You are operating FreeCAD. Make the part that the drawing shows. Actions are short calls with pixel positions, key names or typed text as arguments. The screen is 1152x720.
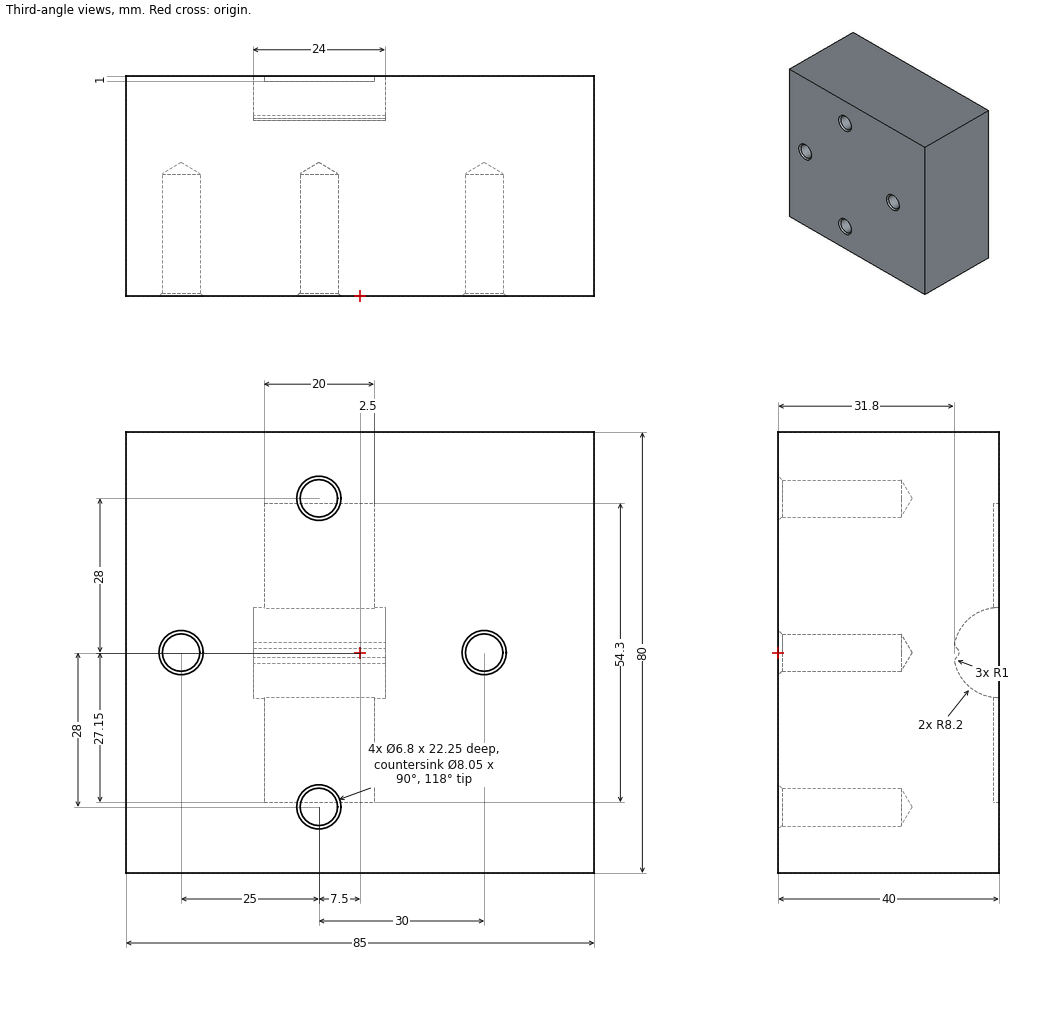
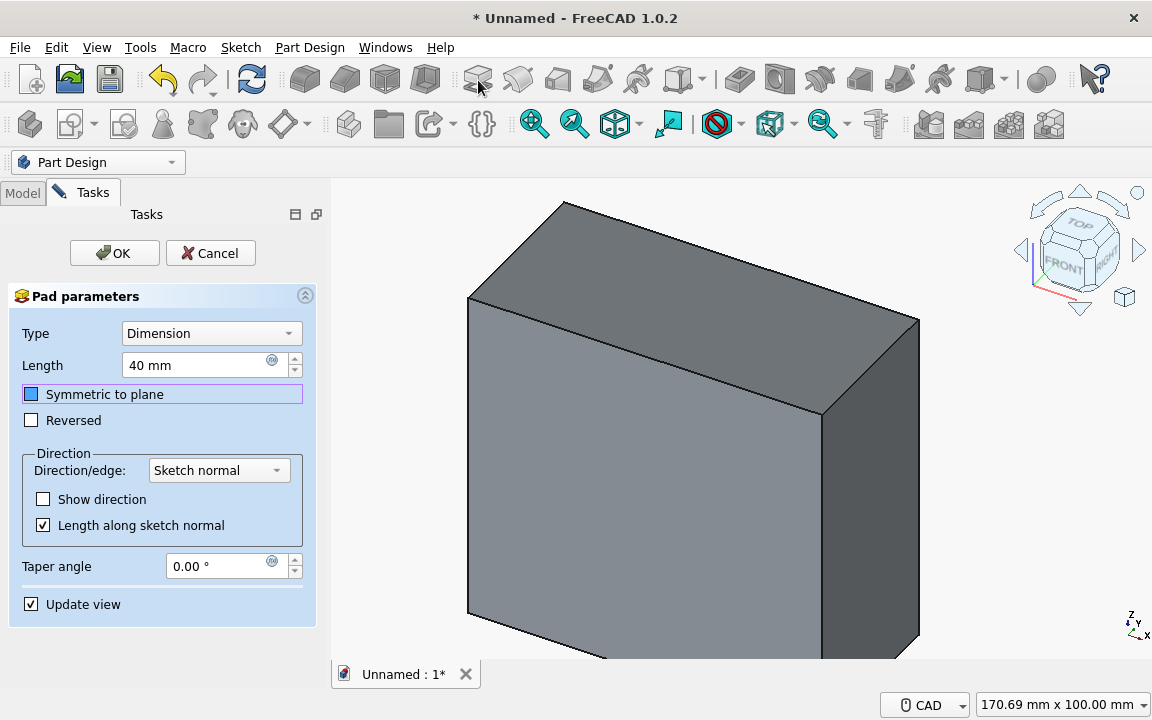
click(30, 420)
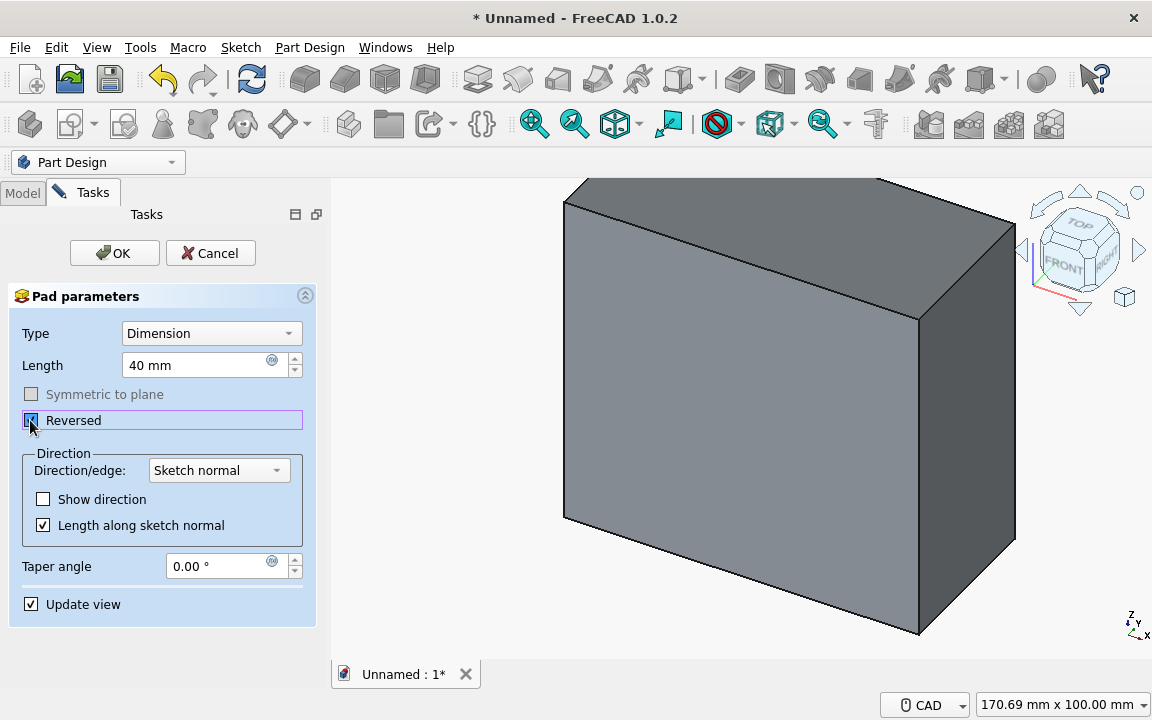
click(115, 253)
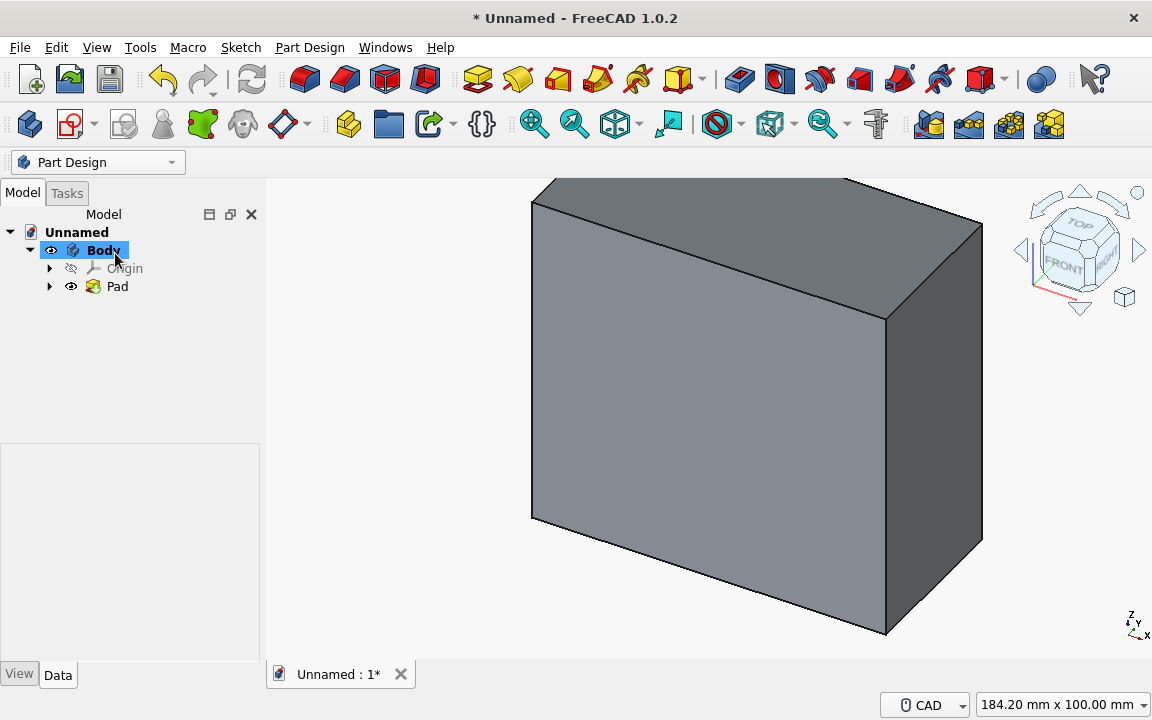
click(536, 124)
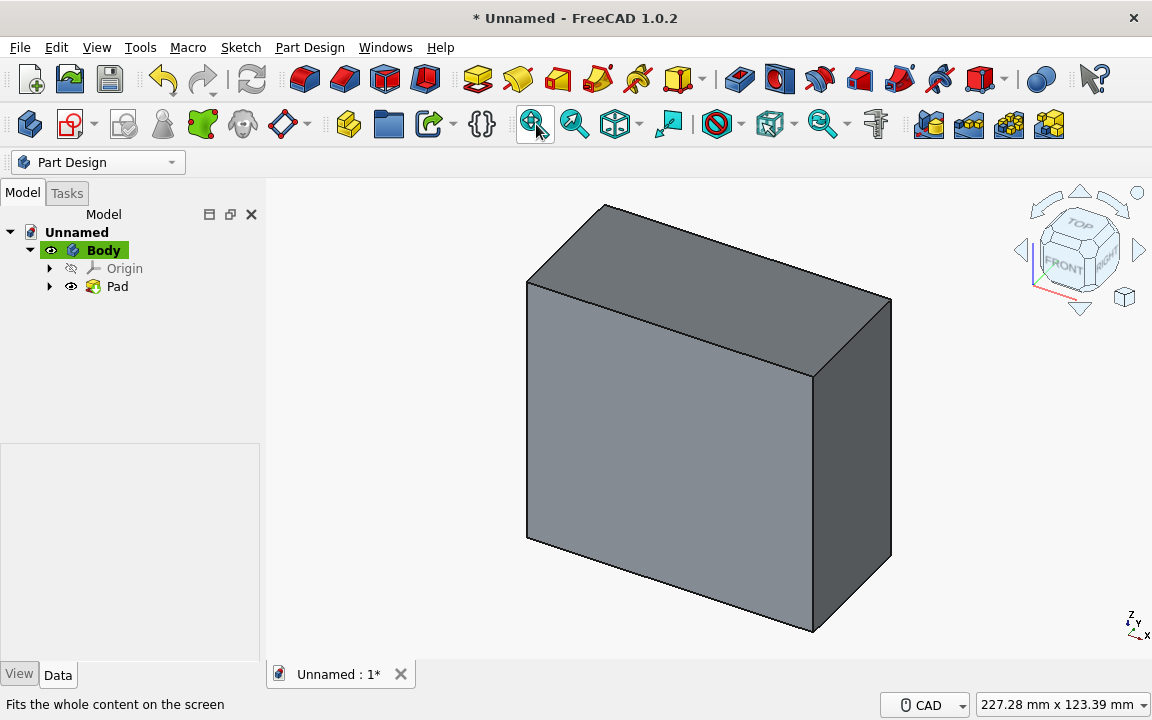
click(670, 456)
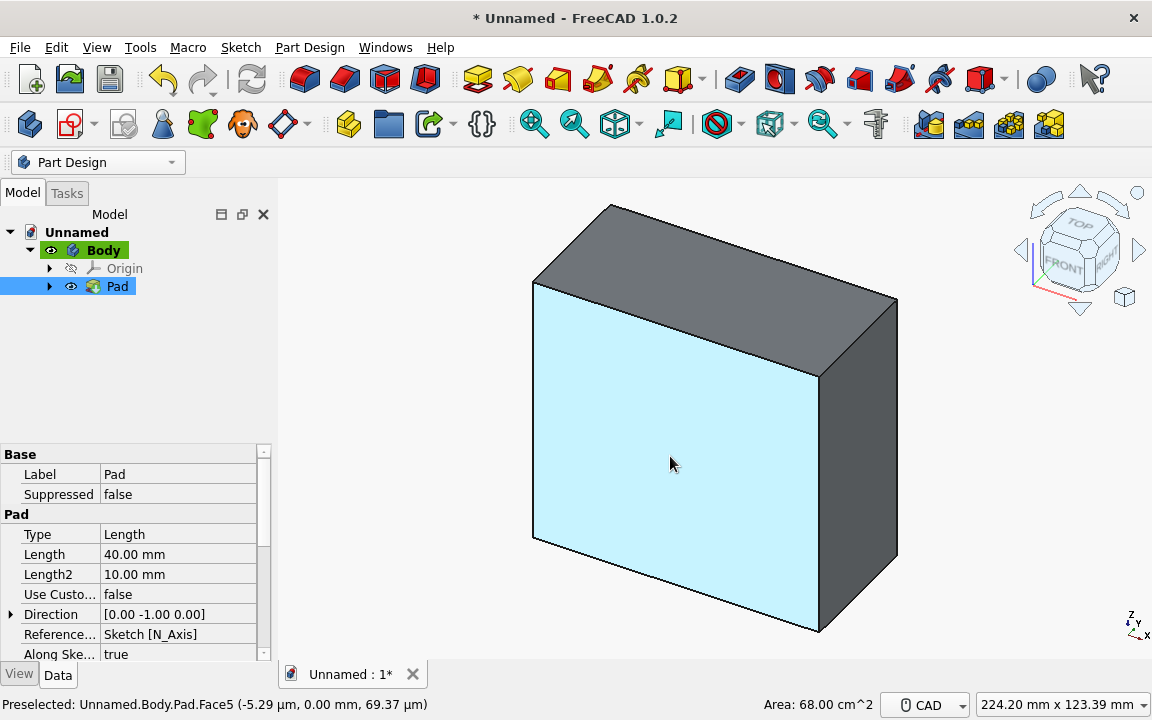
click(70, 124)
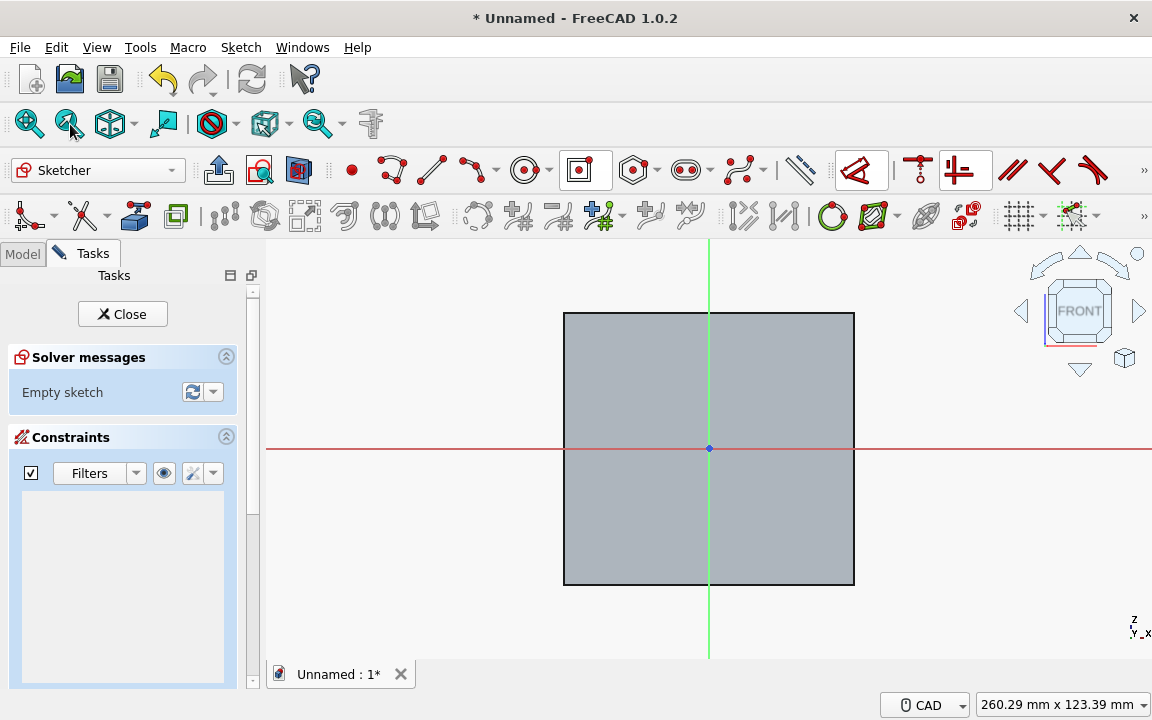
click(526, 170)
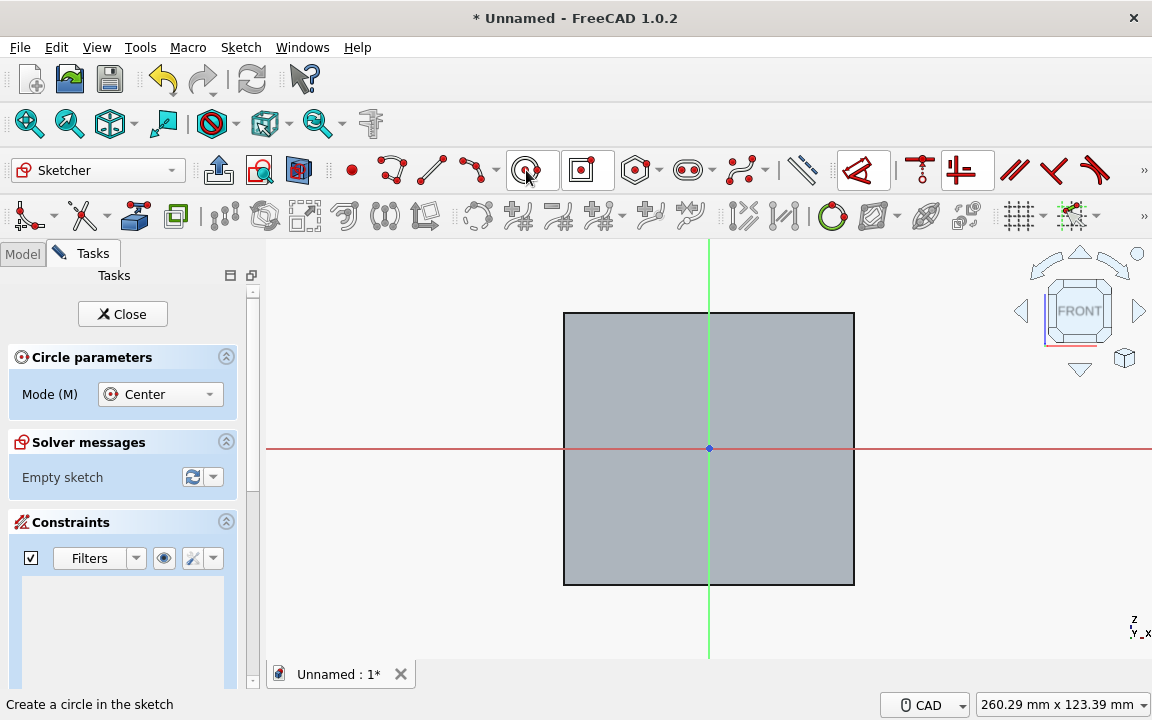
scroll(683, 544, up, 4)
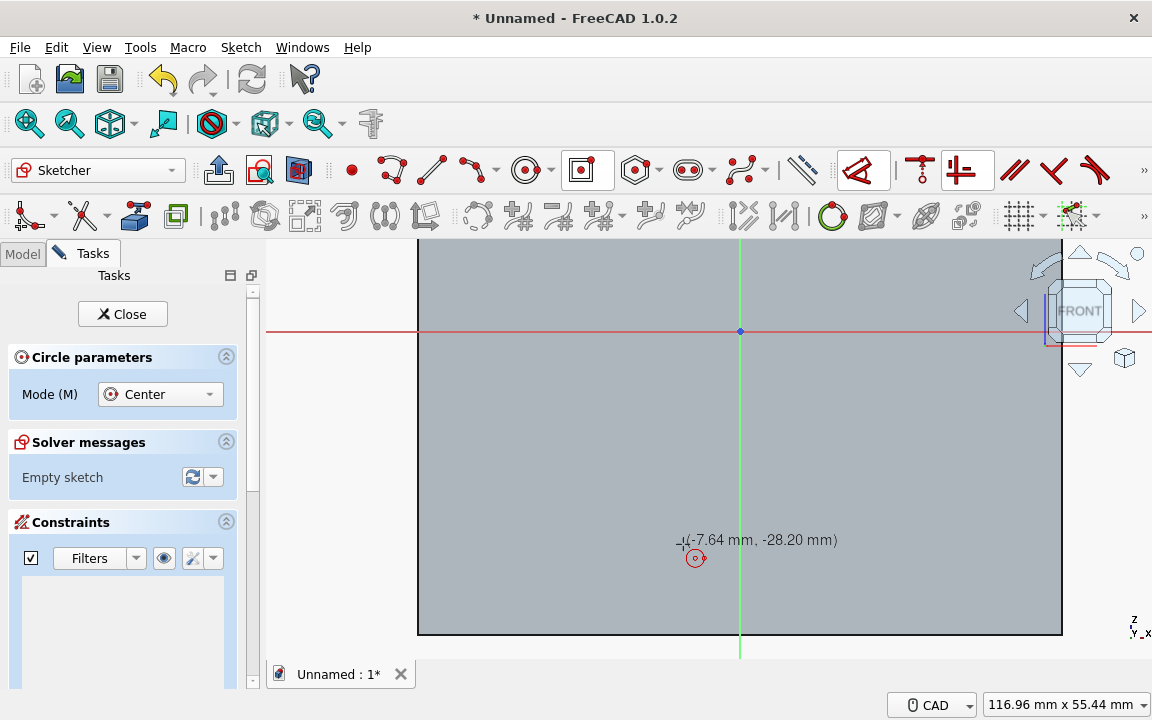
click(683, 544)
move(702, 526)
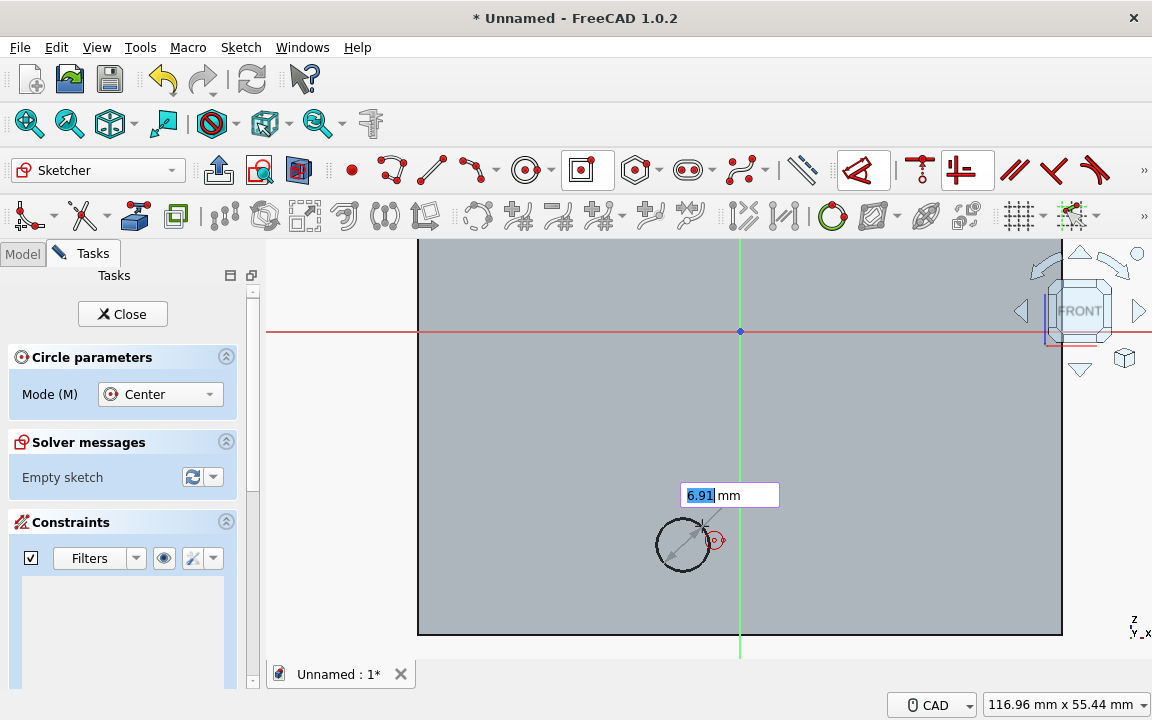
text(6.8)
key(Return)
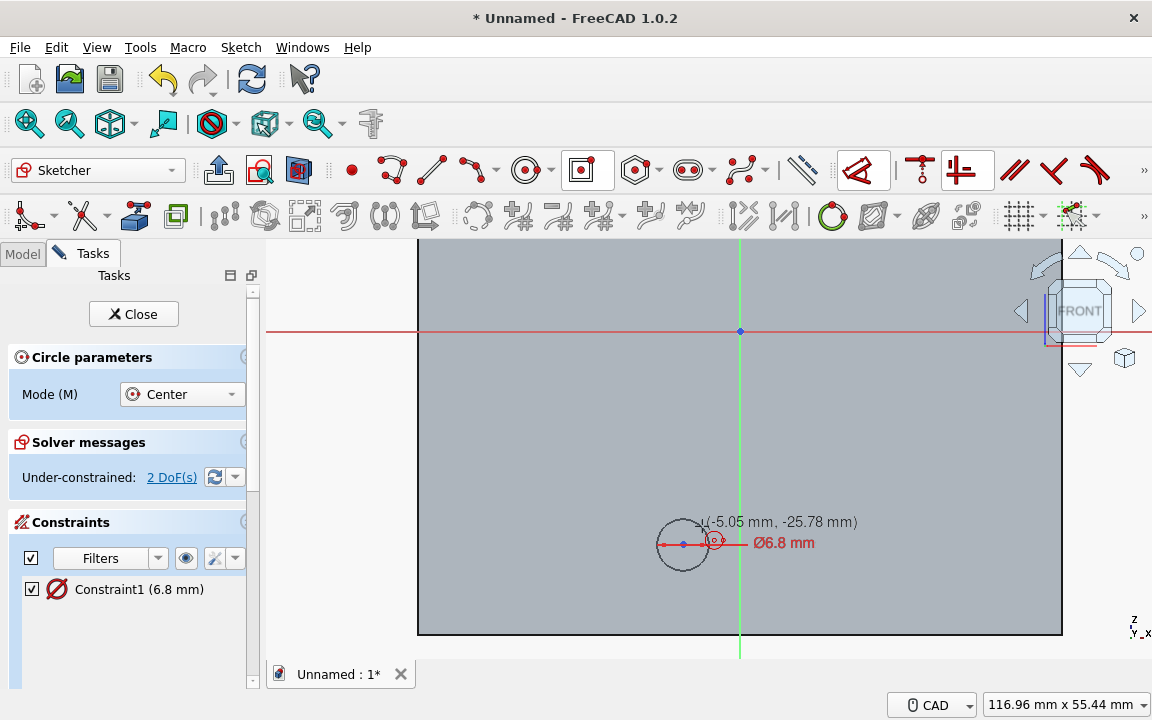
click(911, 332)
move(929, 313)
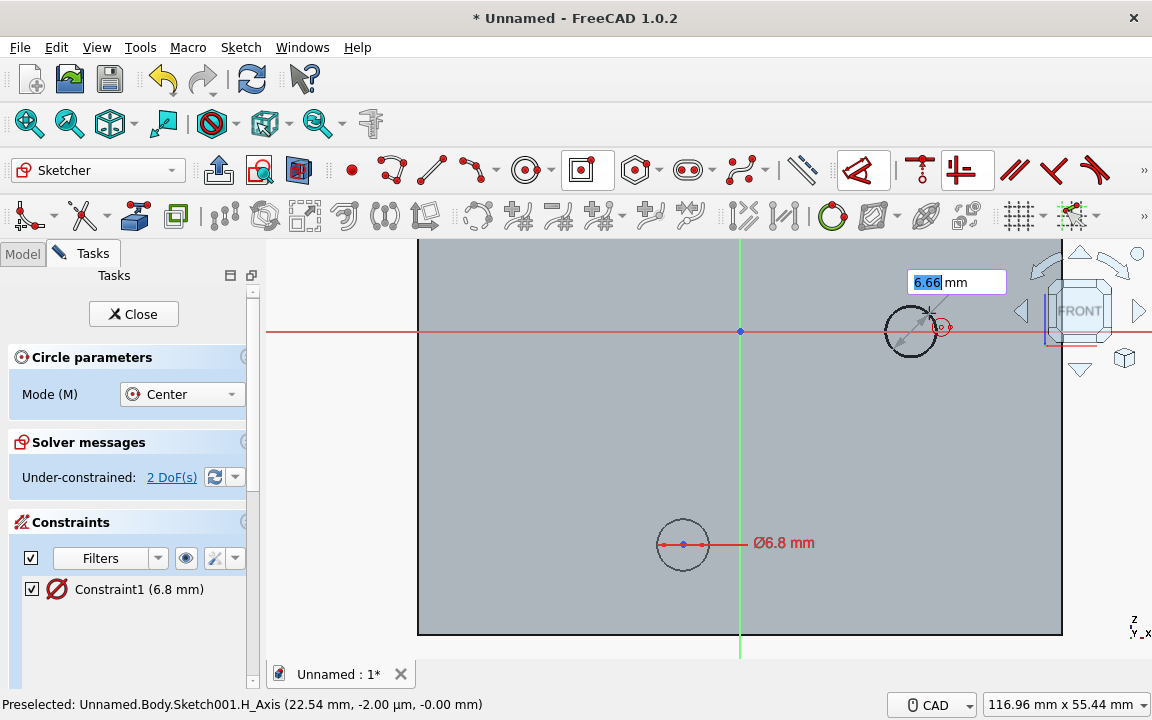
text(6.8)
key(Return)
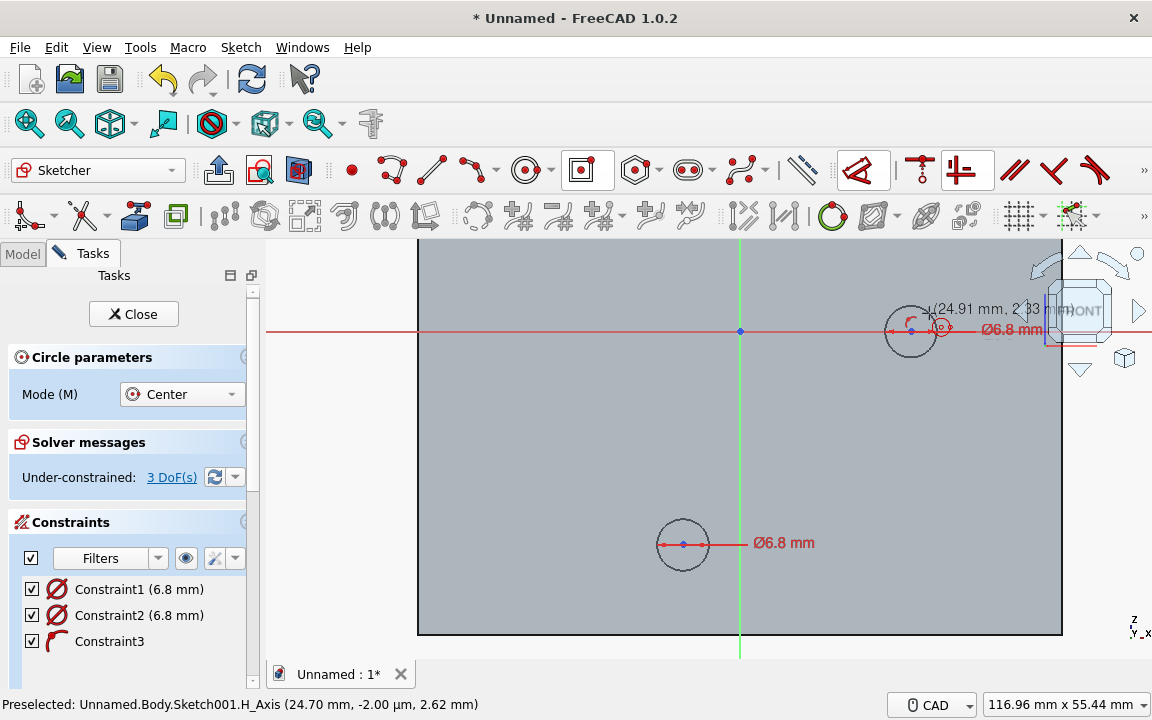
scroll(565, 592, down, 3)